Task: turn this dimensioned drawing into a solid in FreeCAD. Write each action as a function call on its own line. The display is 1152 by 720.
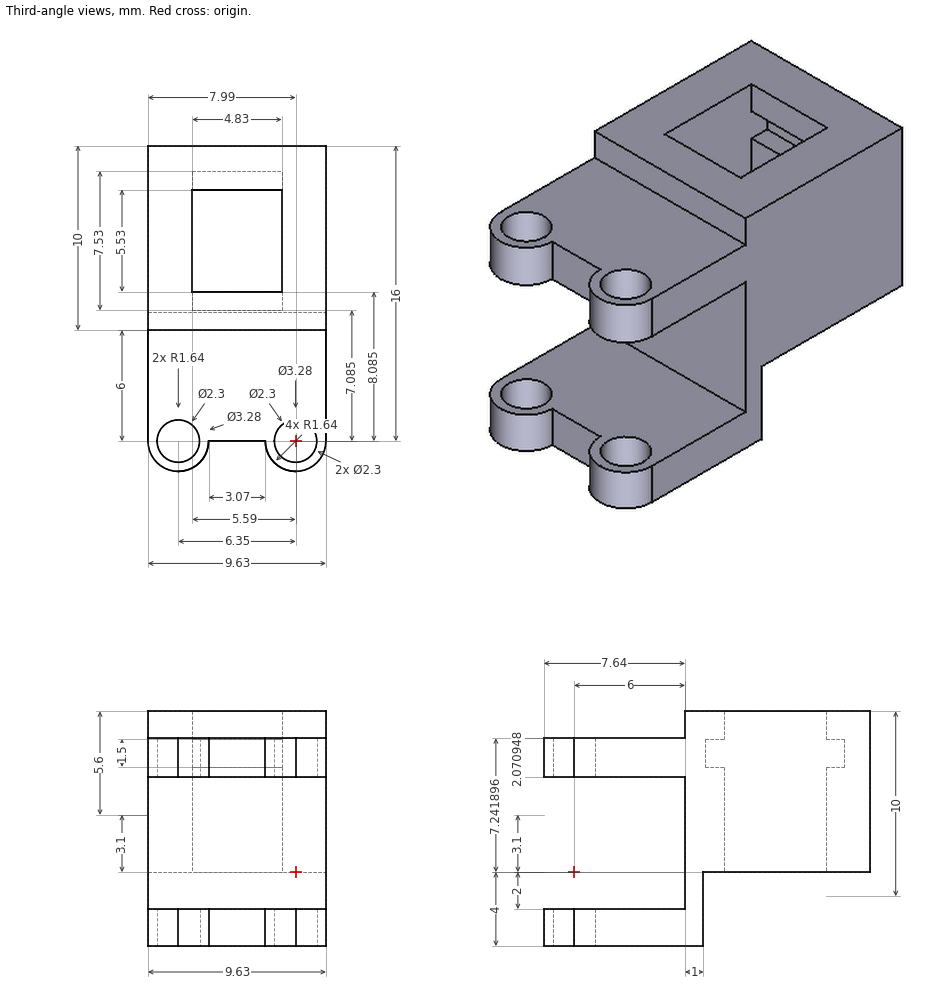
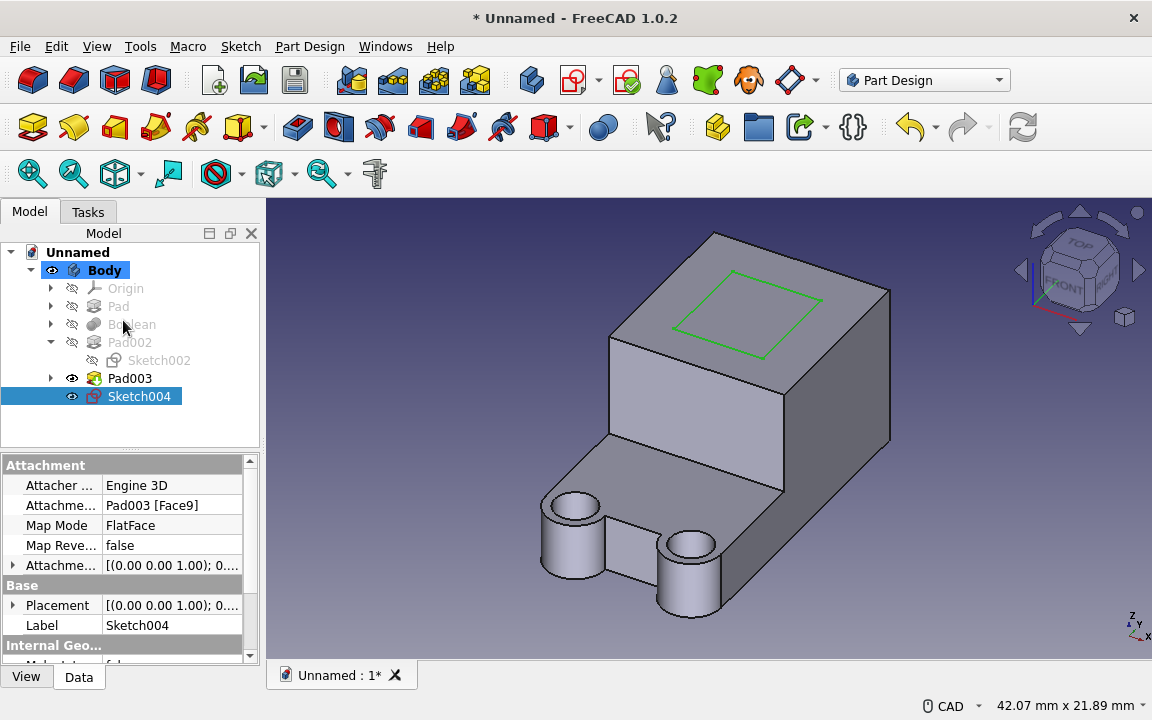
click(298, 128)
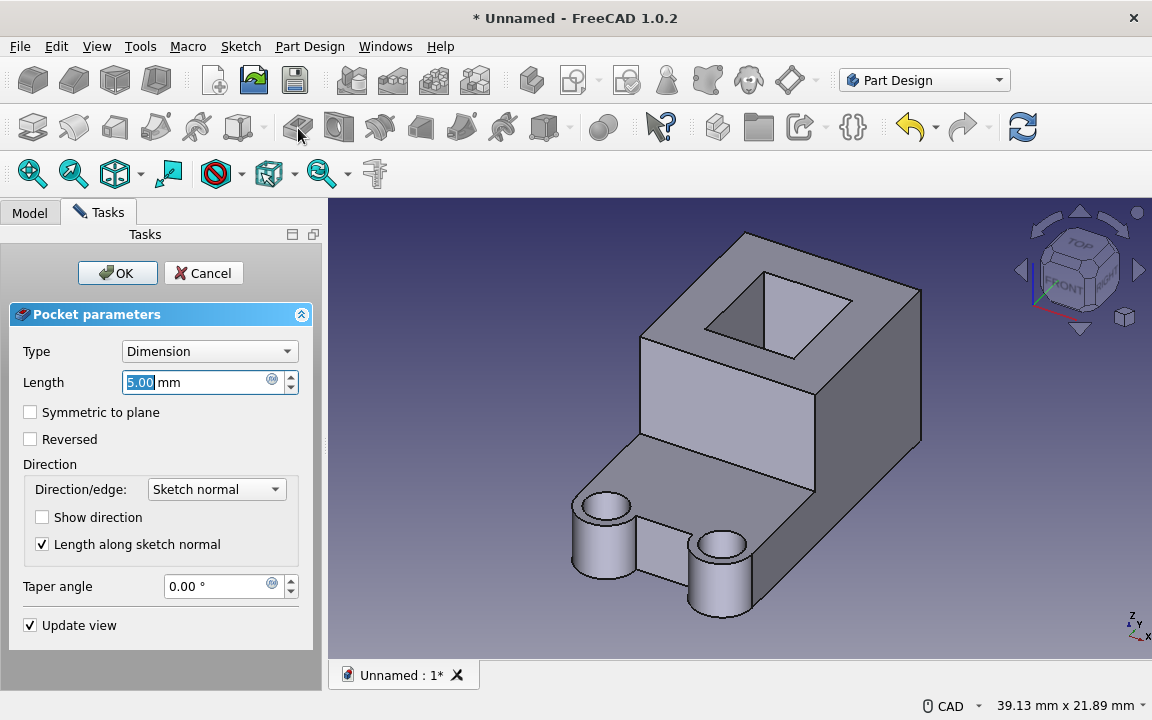
text(10)
key(Tab)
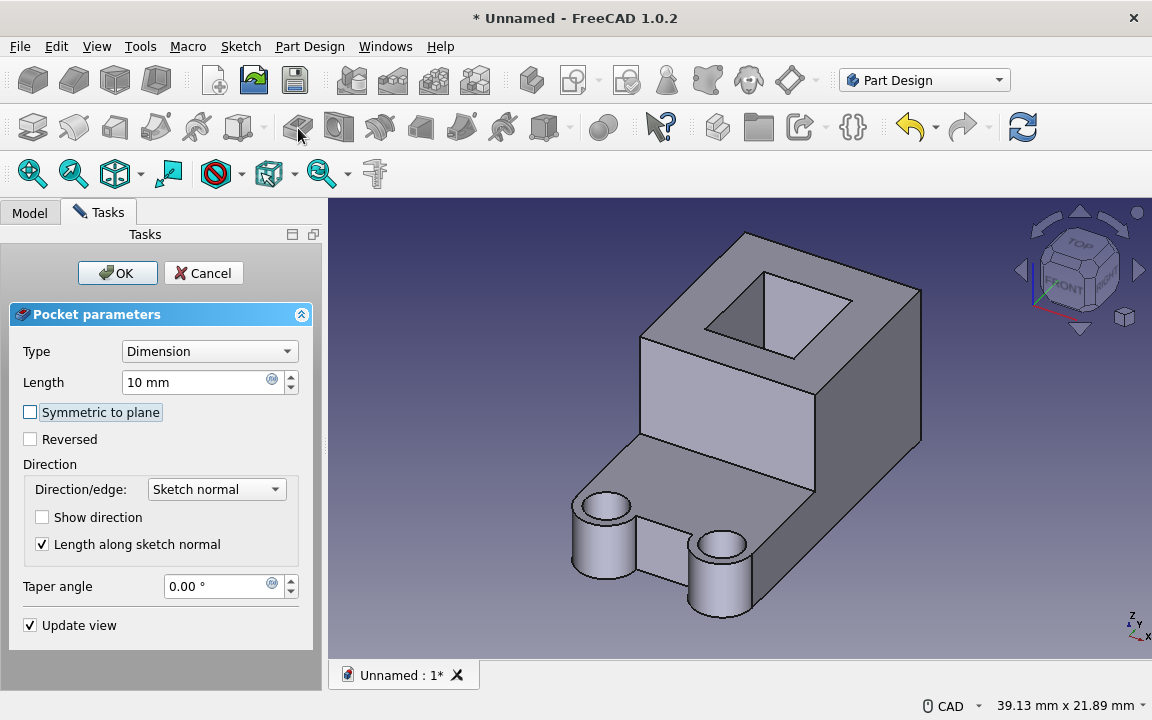
click(118, 273)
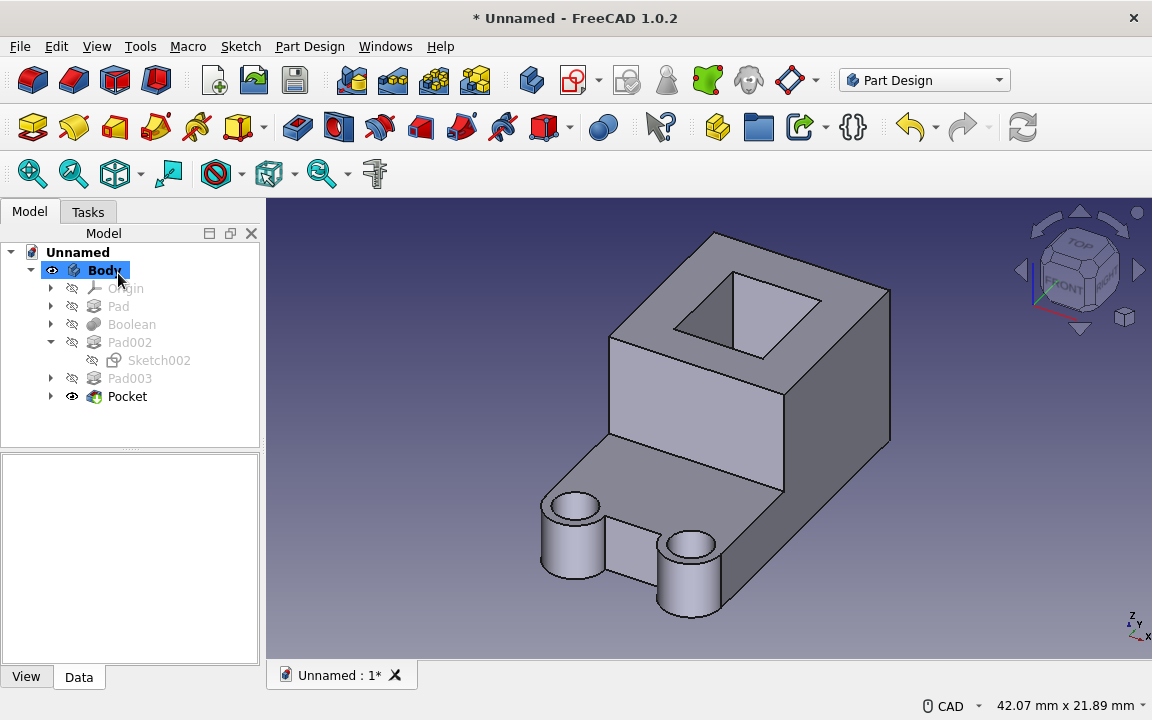
click(51, 288)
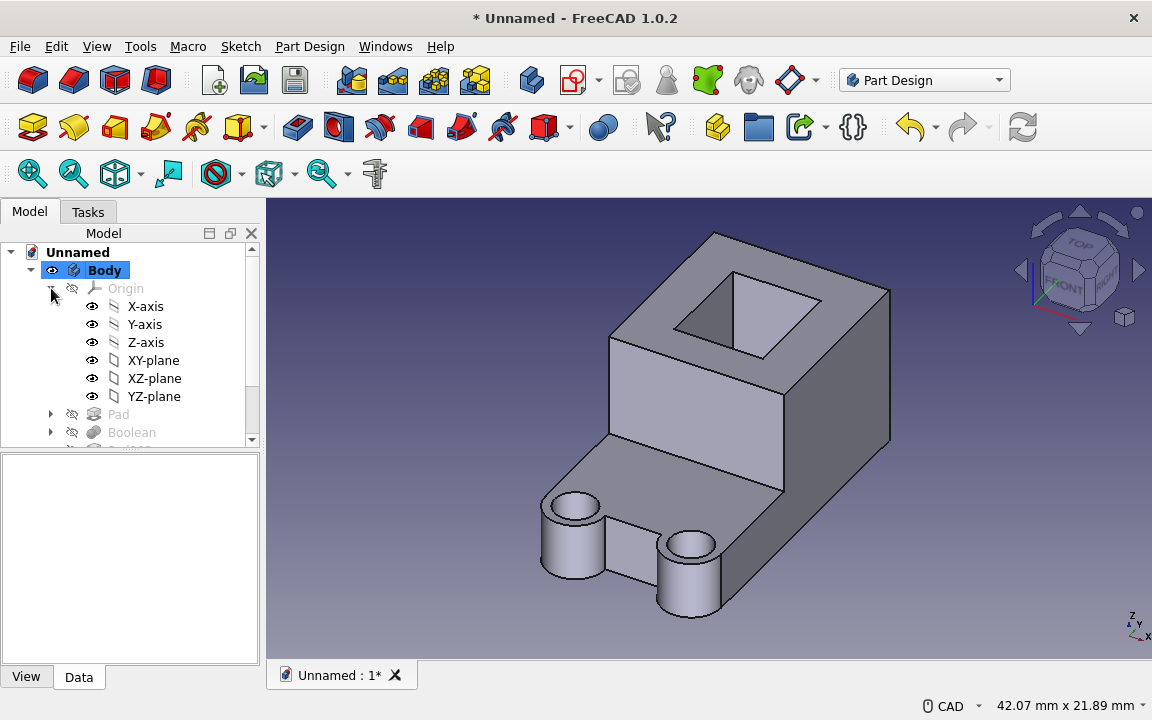
click(137, 360)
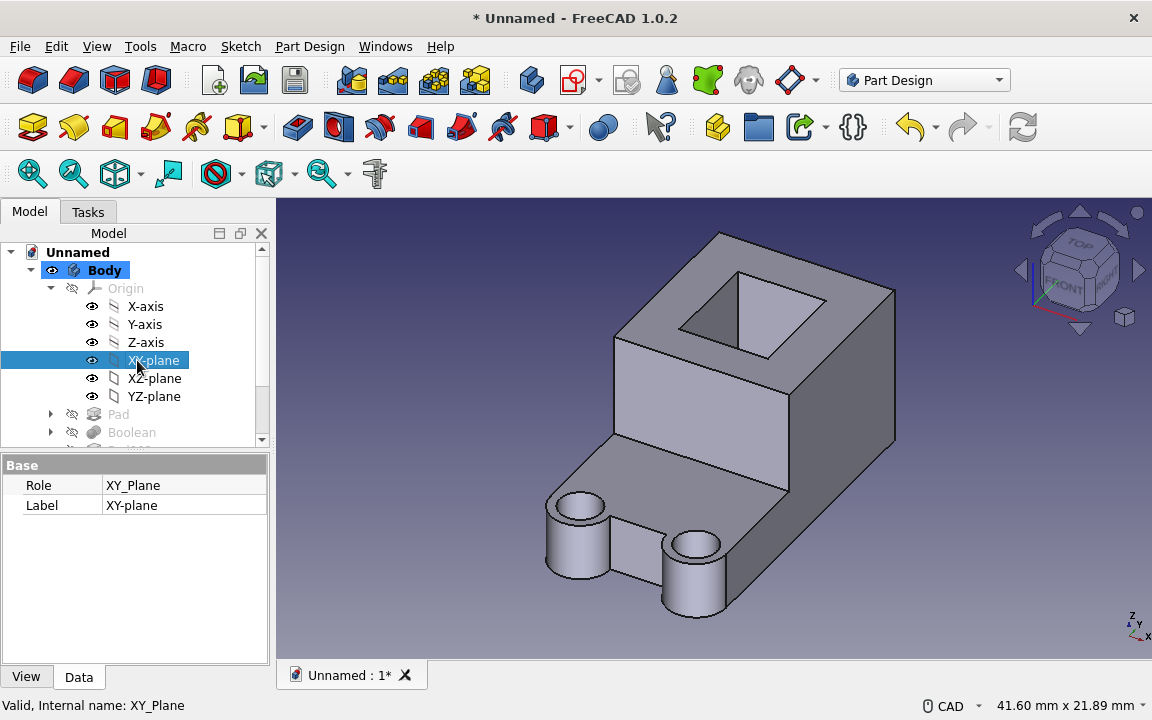
click(790, 80)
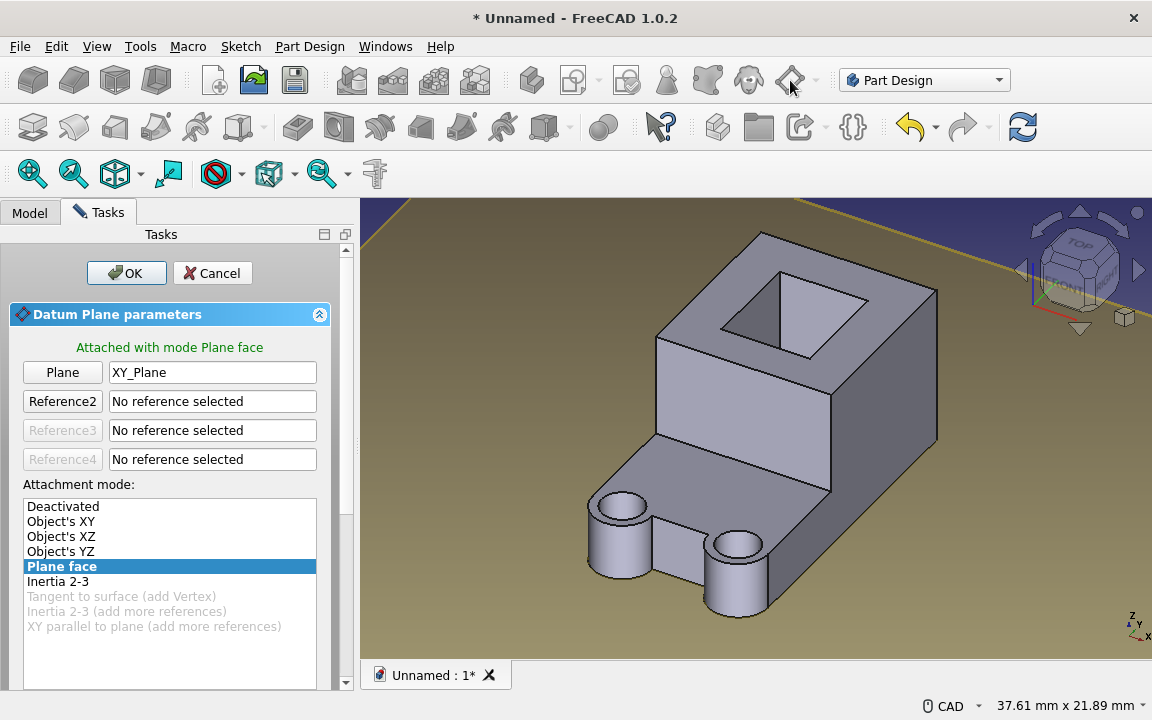
scroll(346, 467, down, 4)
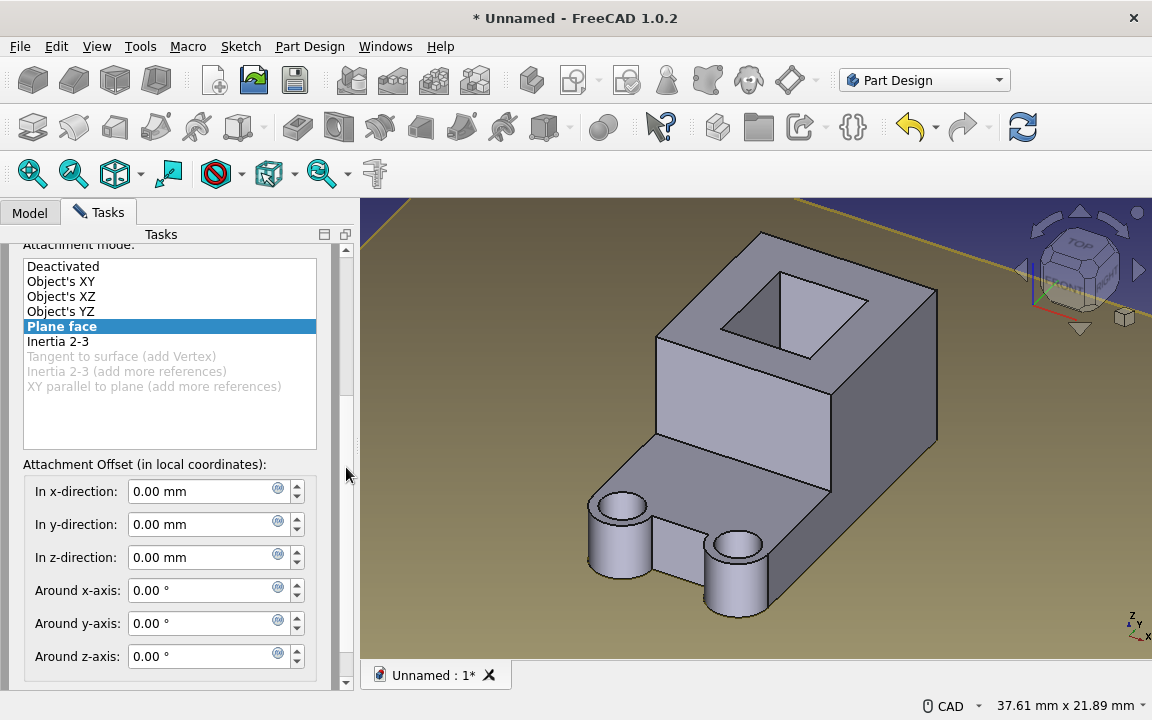
triple_click(210, 558)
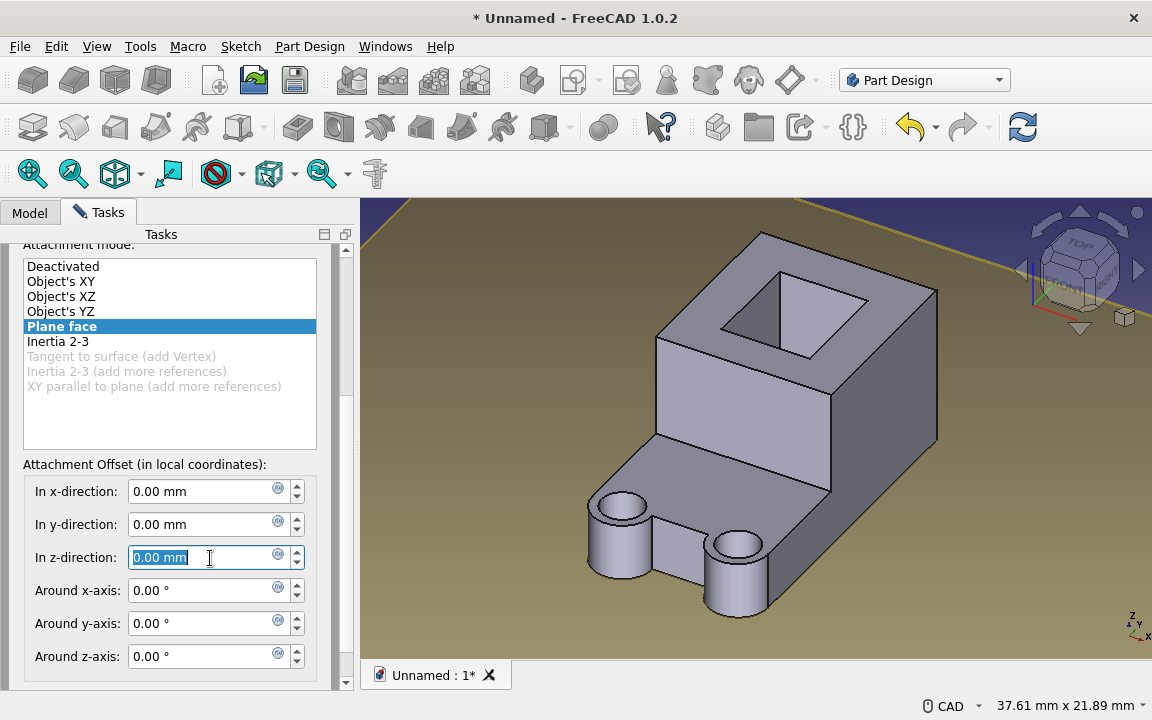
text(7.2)
key(Tab)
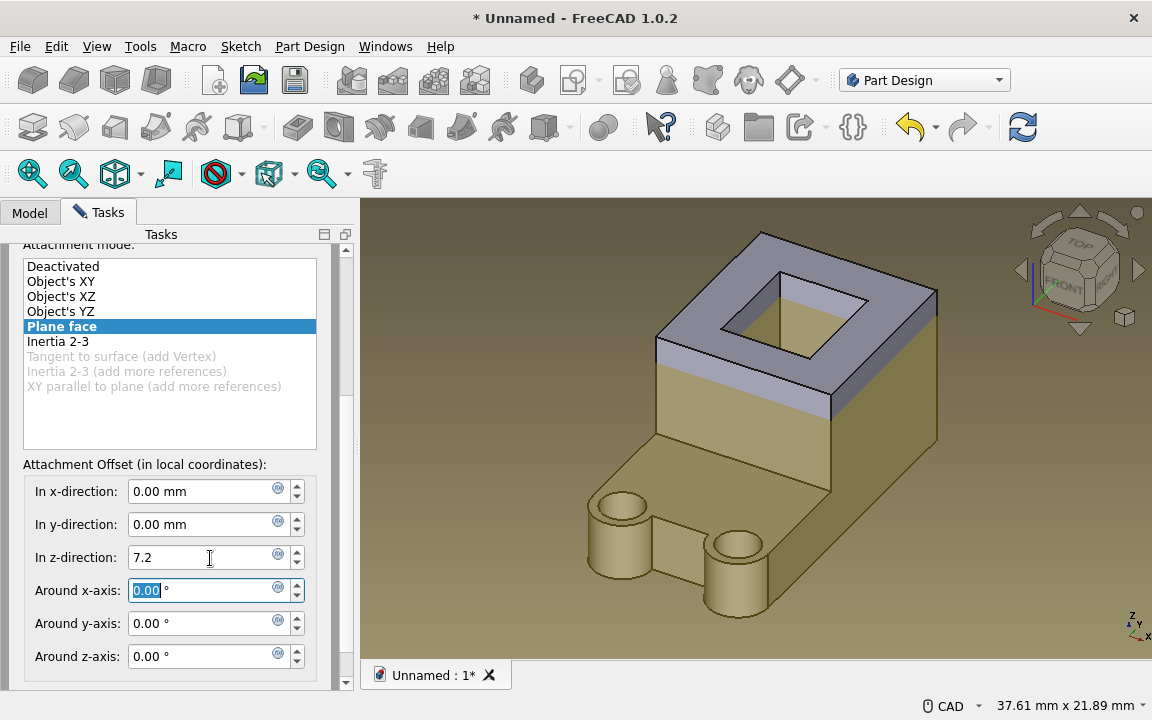
scroll(346, 467, up, 5)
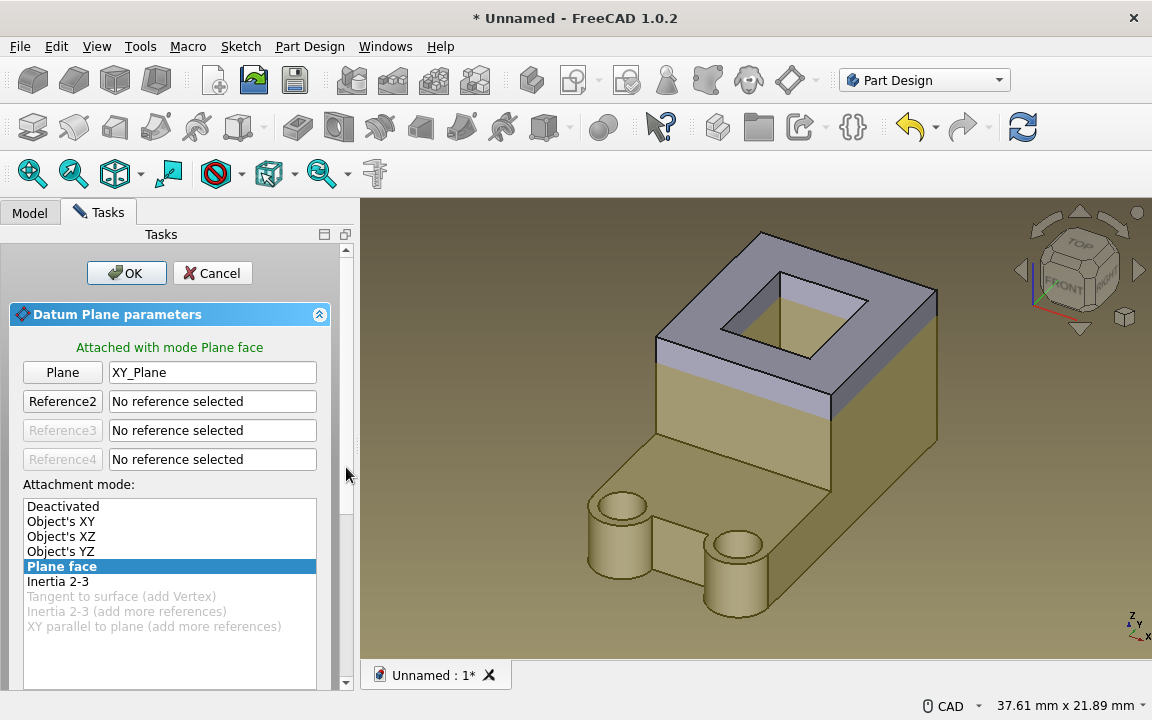
click(127, 273)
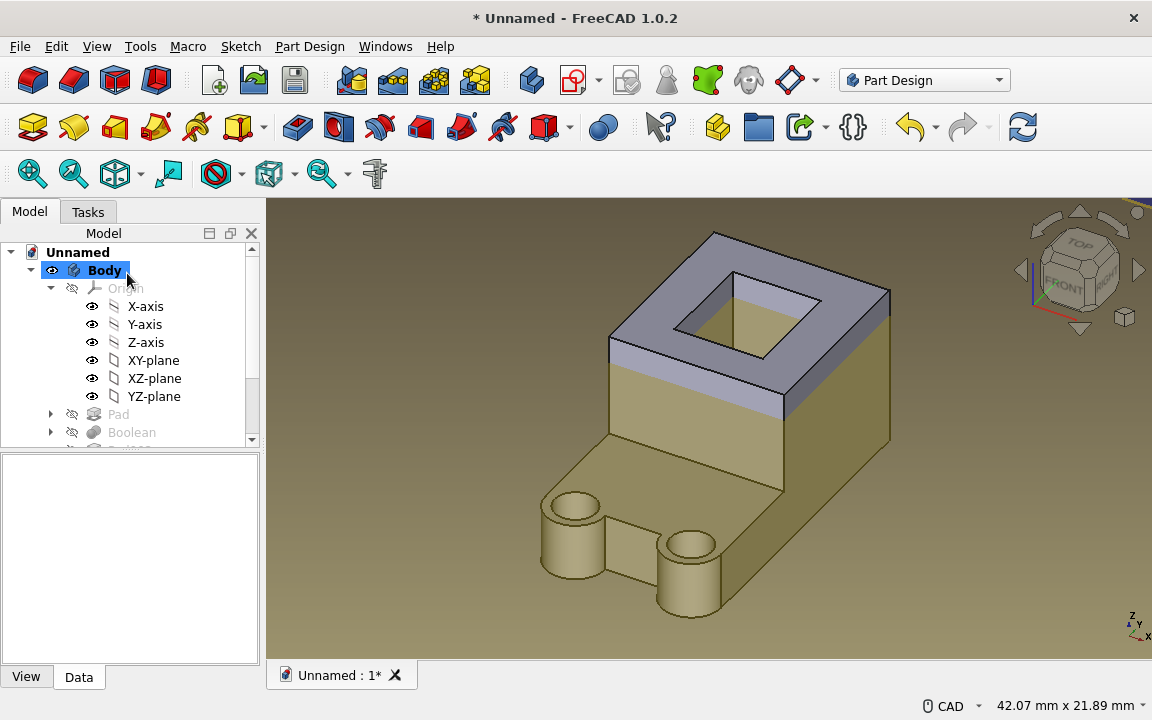
scroll(101, 338, down, 3)